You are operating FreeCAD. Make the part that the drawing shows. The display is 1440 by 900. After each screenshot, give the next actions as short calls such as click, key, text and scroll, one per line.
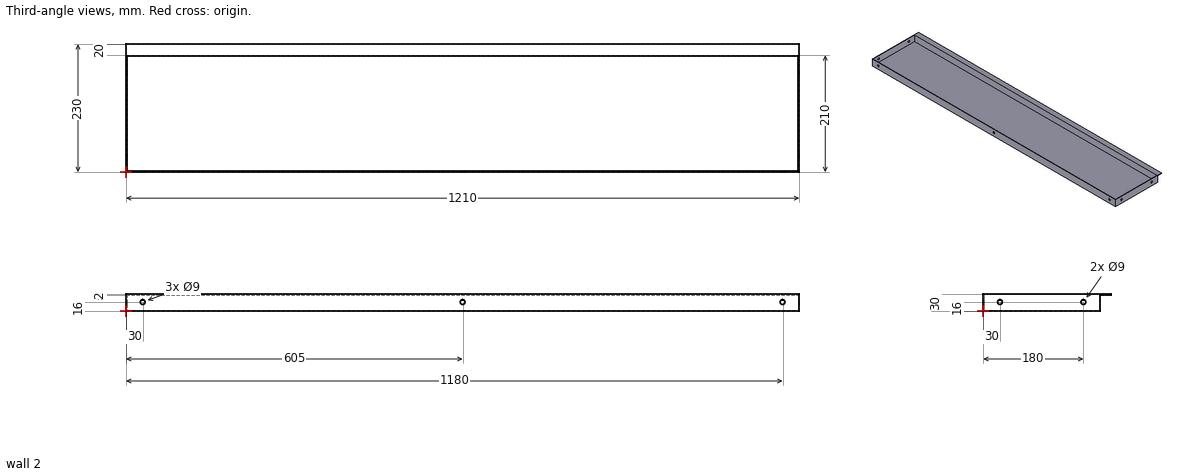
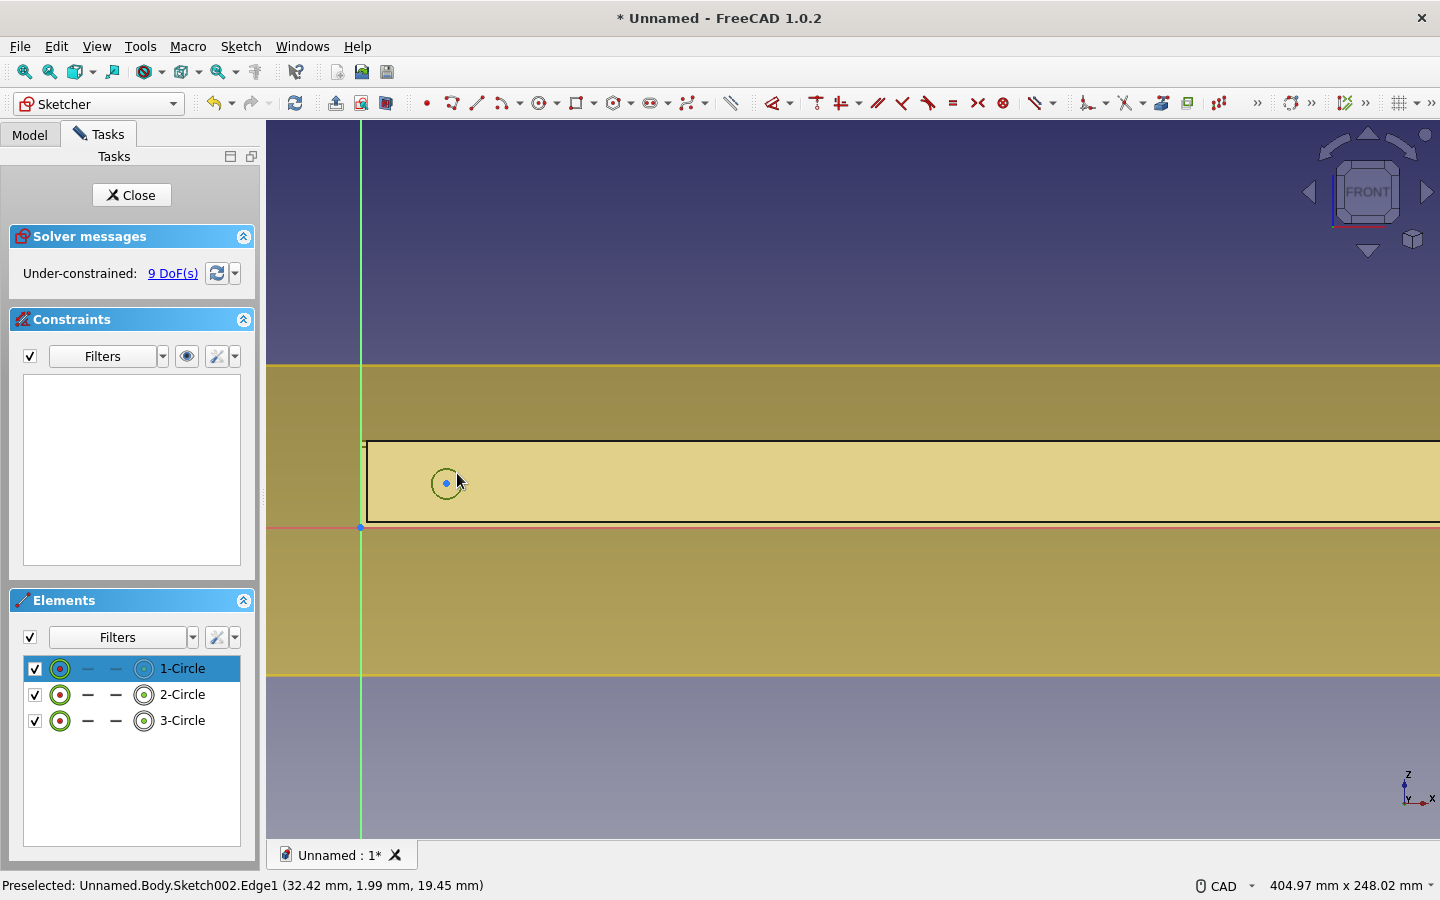
scroll(457, 475, down, 8)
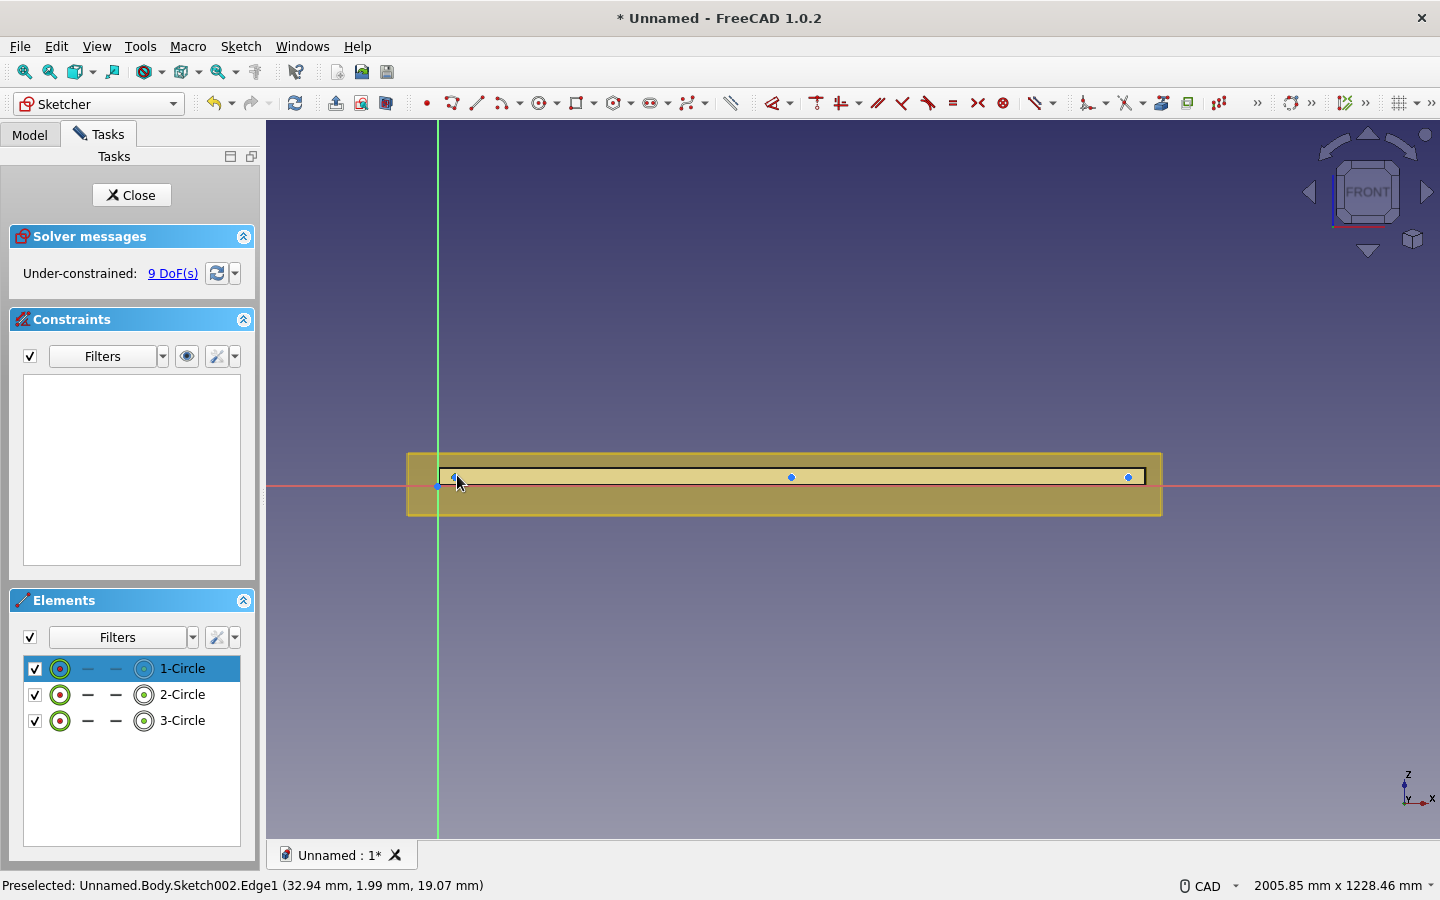
scroll(1130, 475, up, 8)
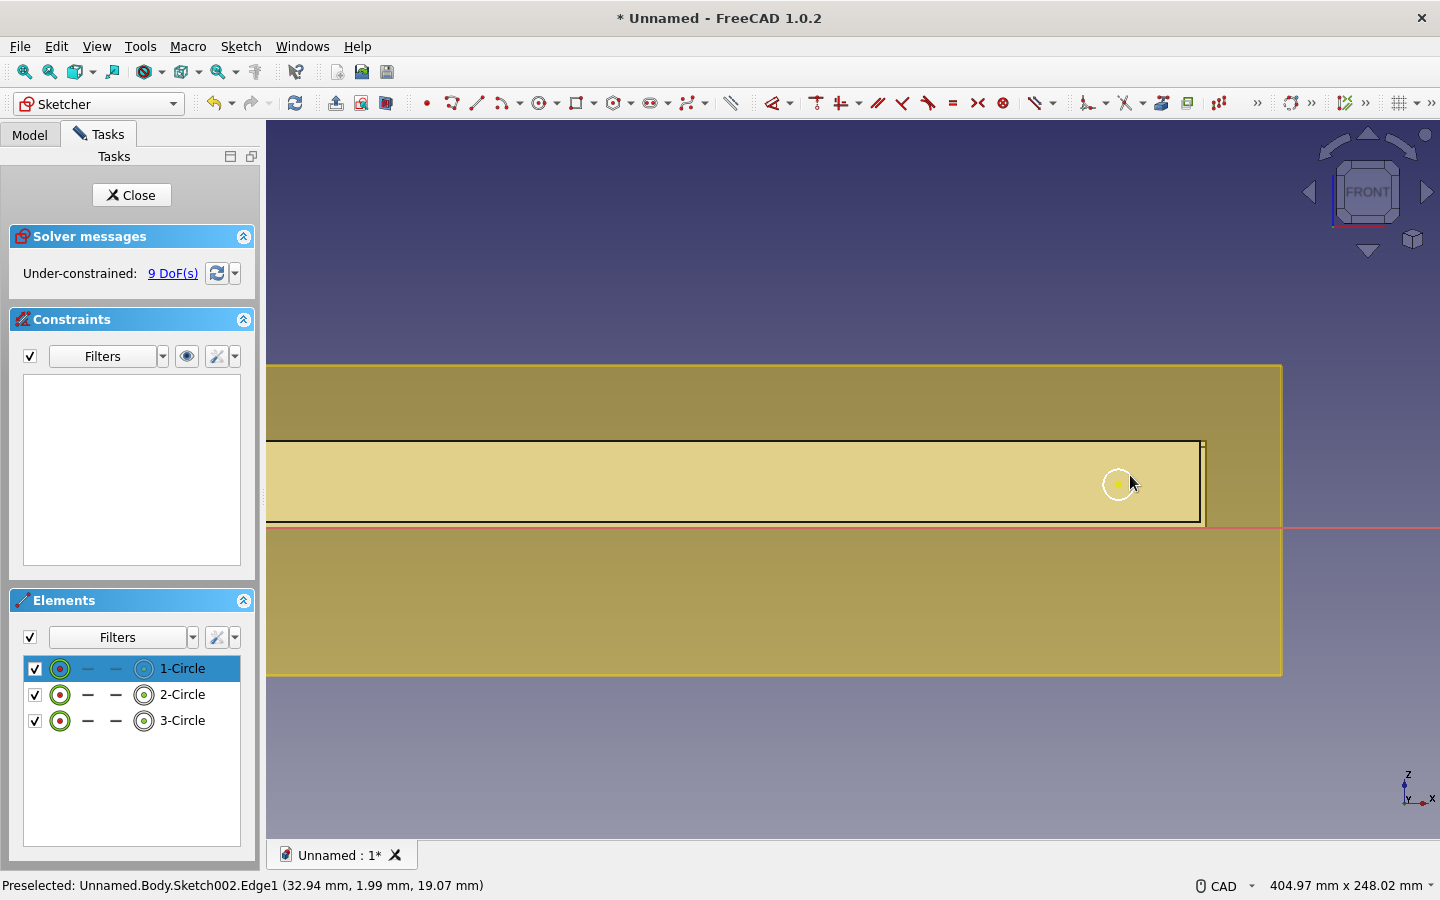
click(1129, 474)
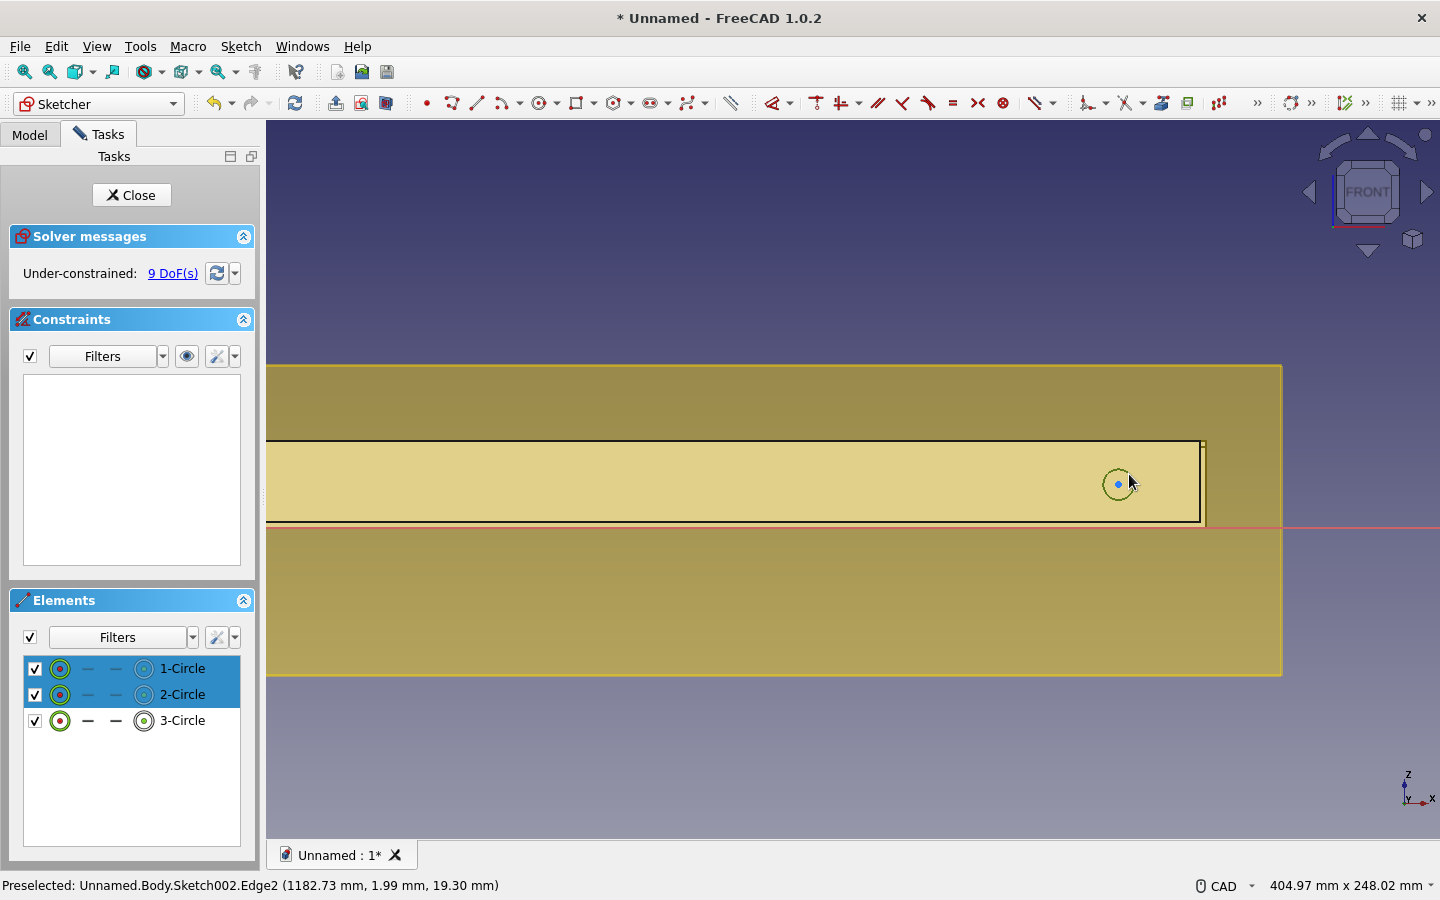
scroll(1131, 475, down, 8)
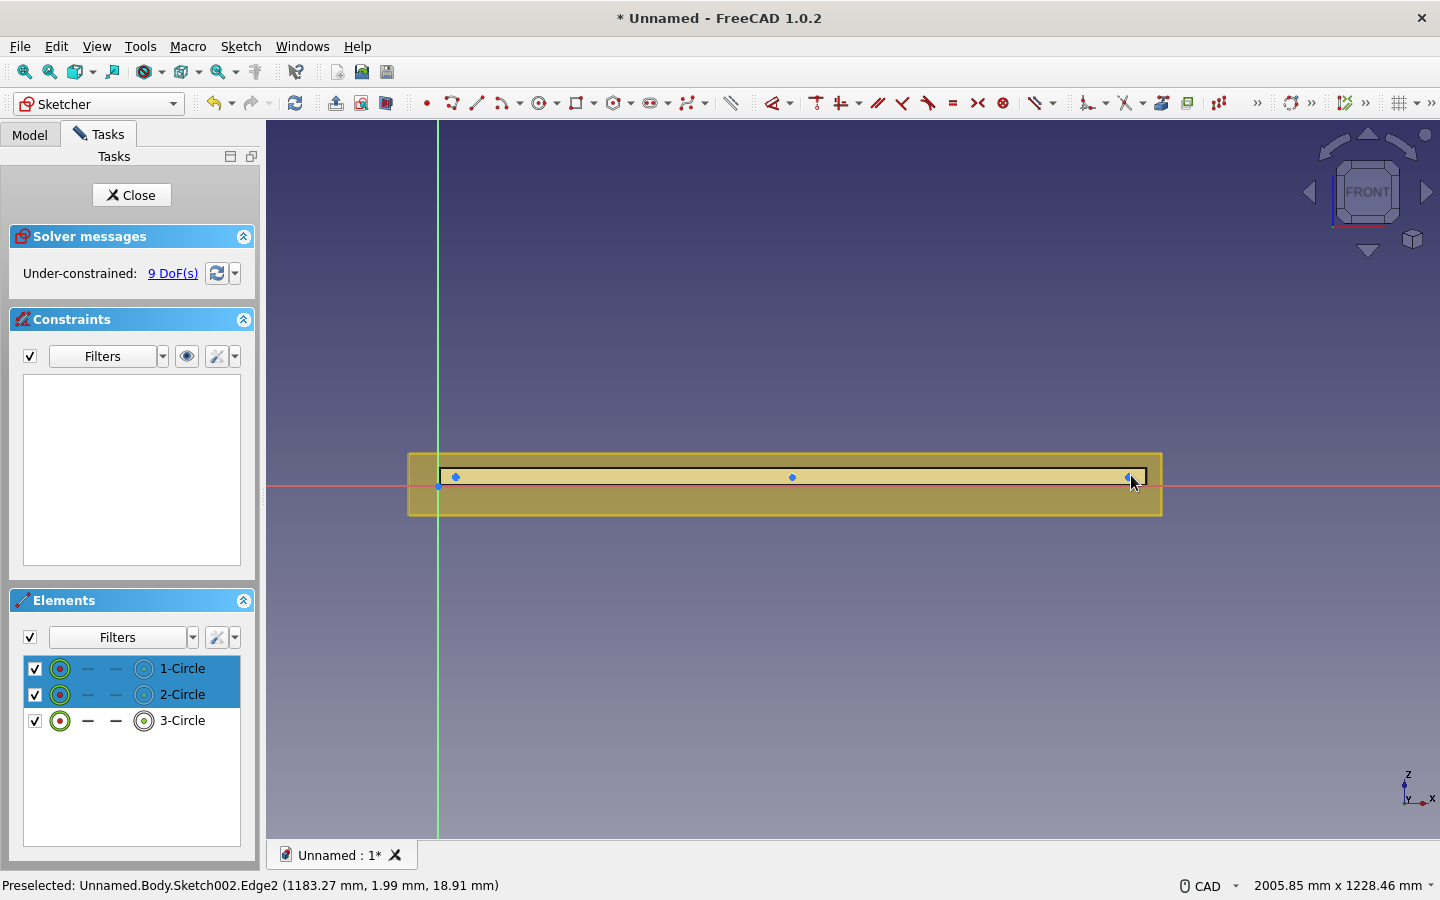
scroll(795, 475, up, 9)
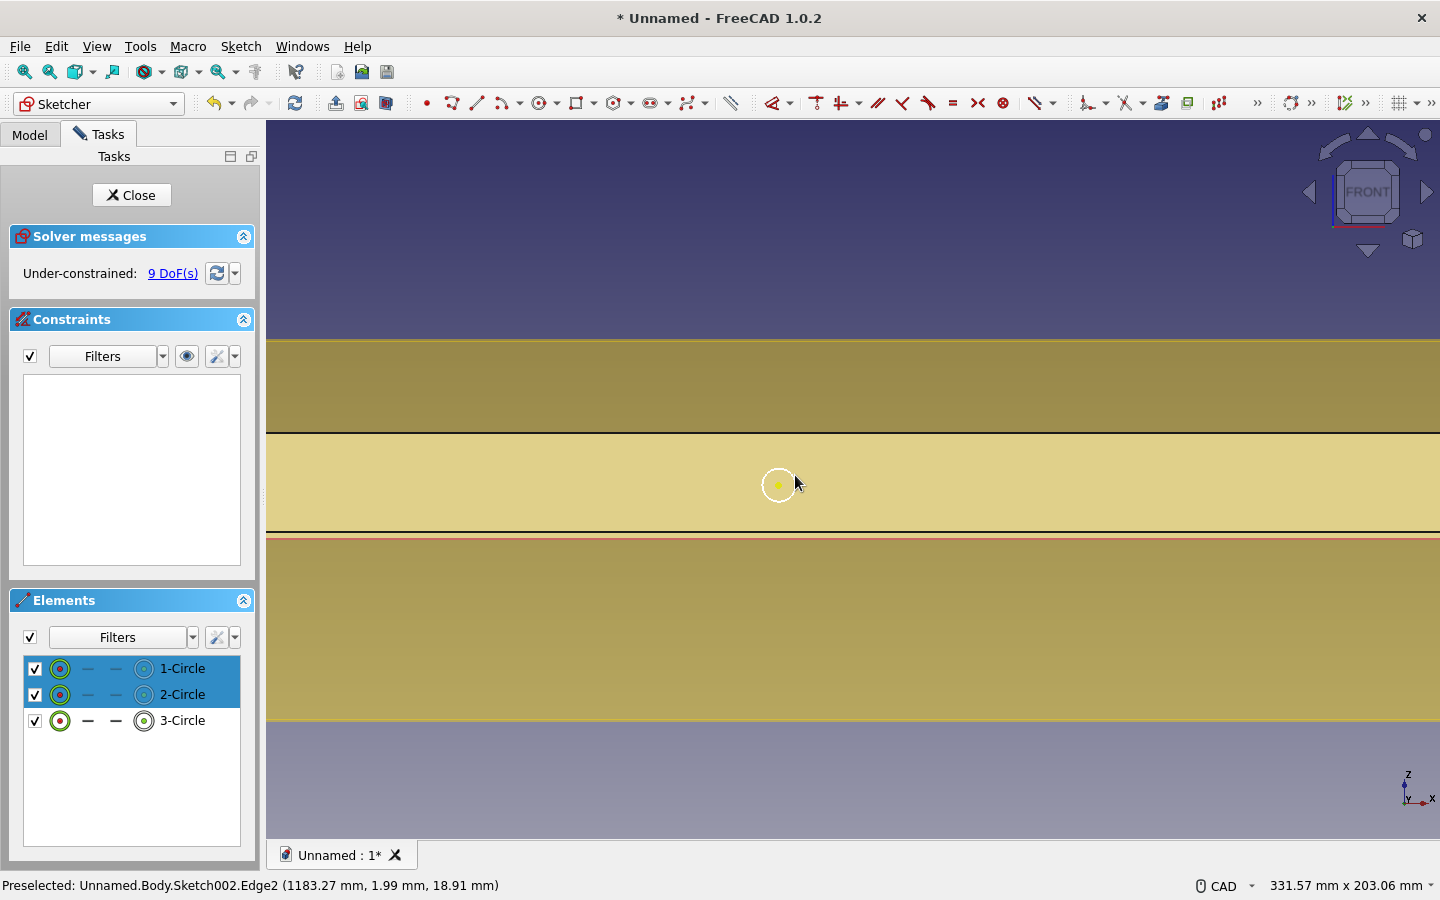
click(791, 473)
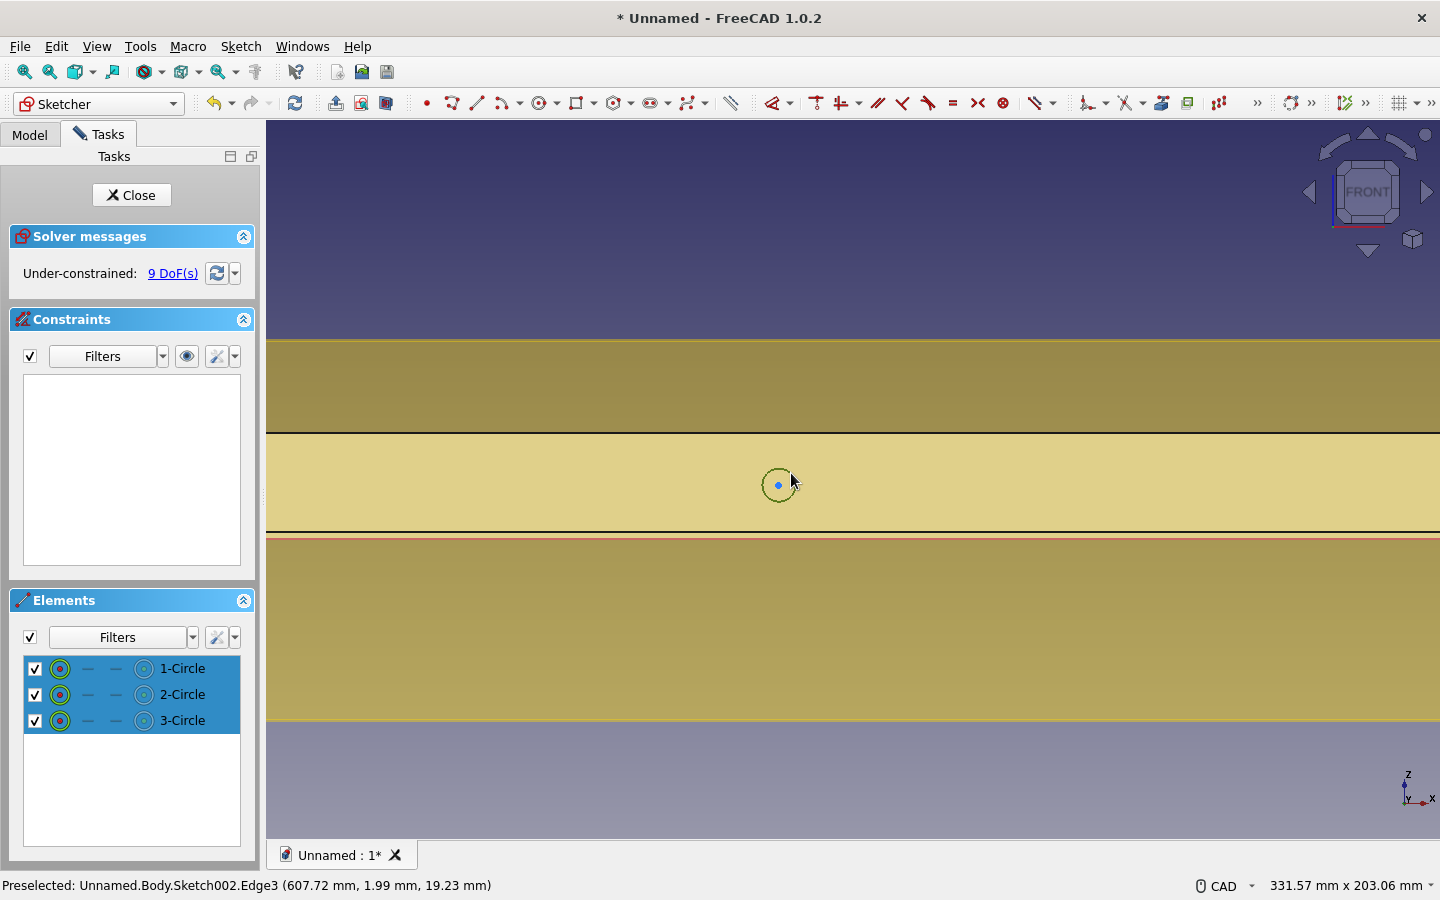
click(953, 104)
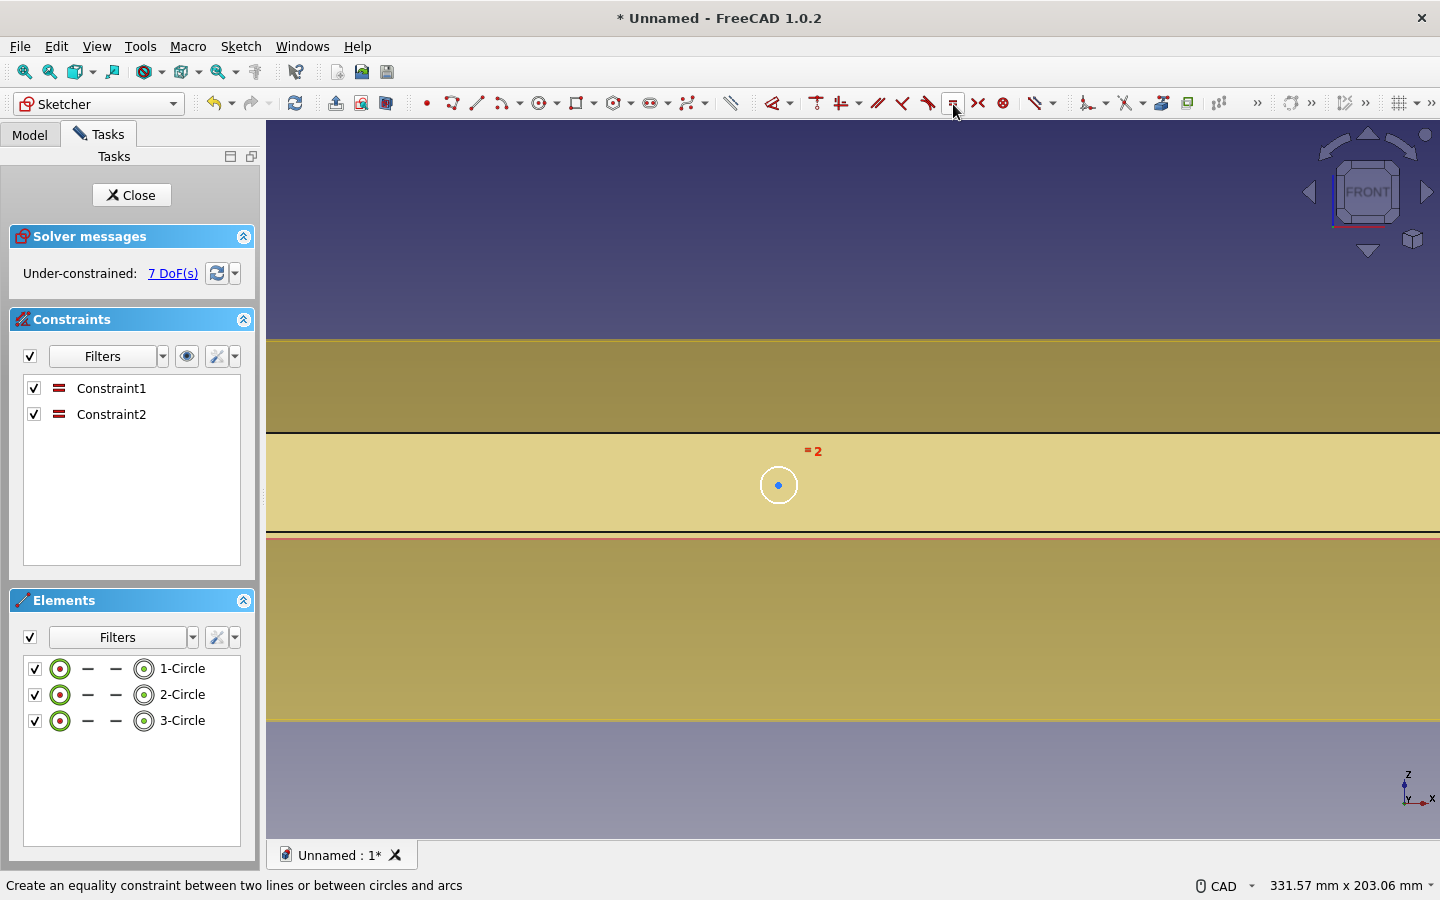
scroll(795, 475, down, 9)